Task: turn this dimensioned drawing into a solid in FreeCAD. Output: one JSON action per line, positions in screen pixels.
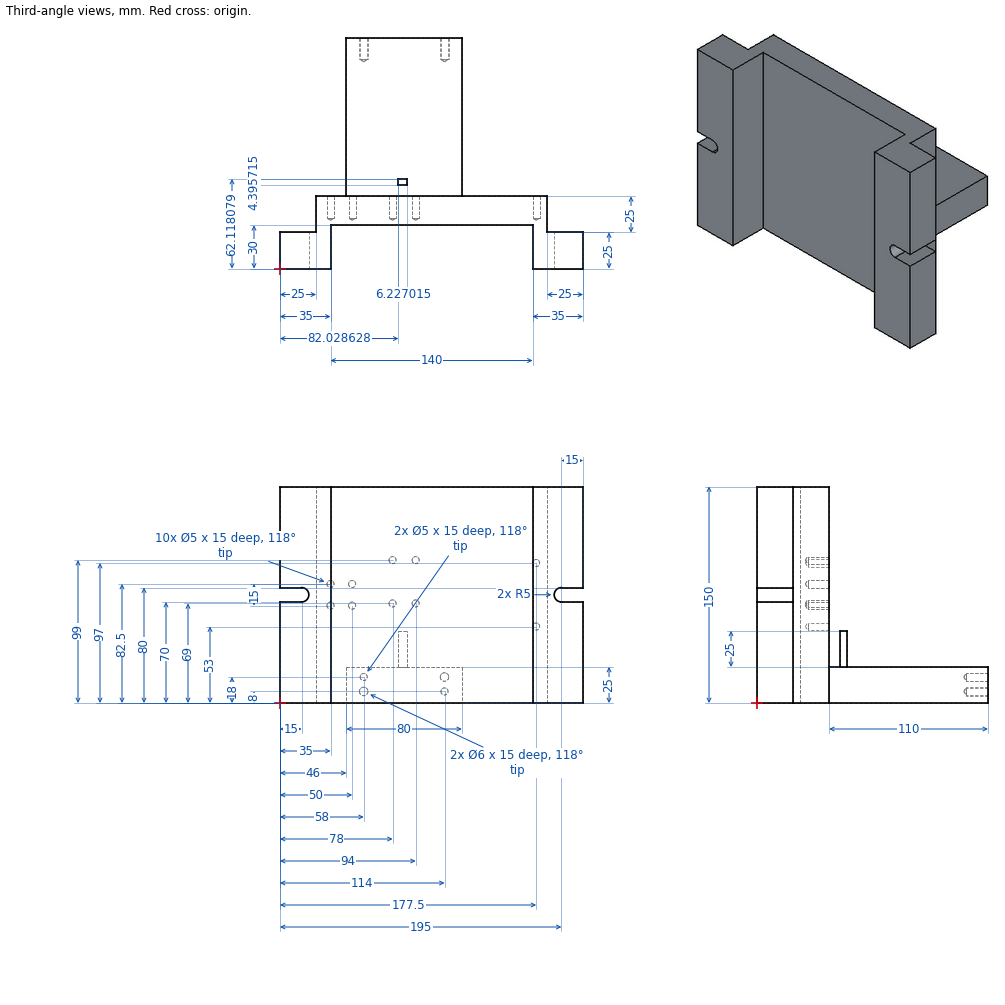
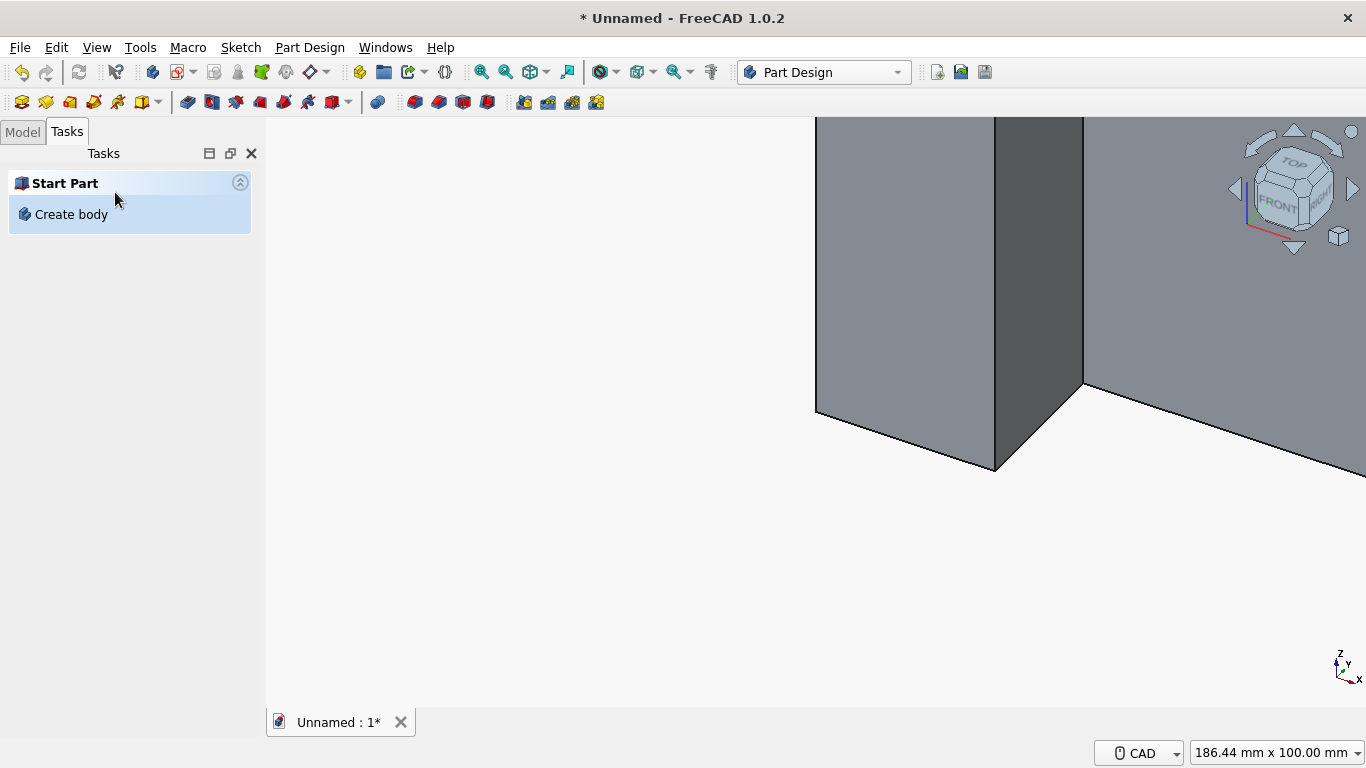
{"action": "left_click", "coordinate": [482, 72]}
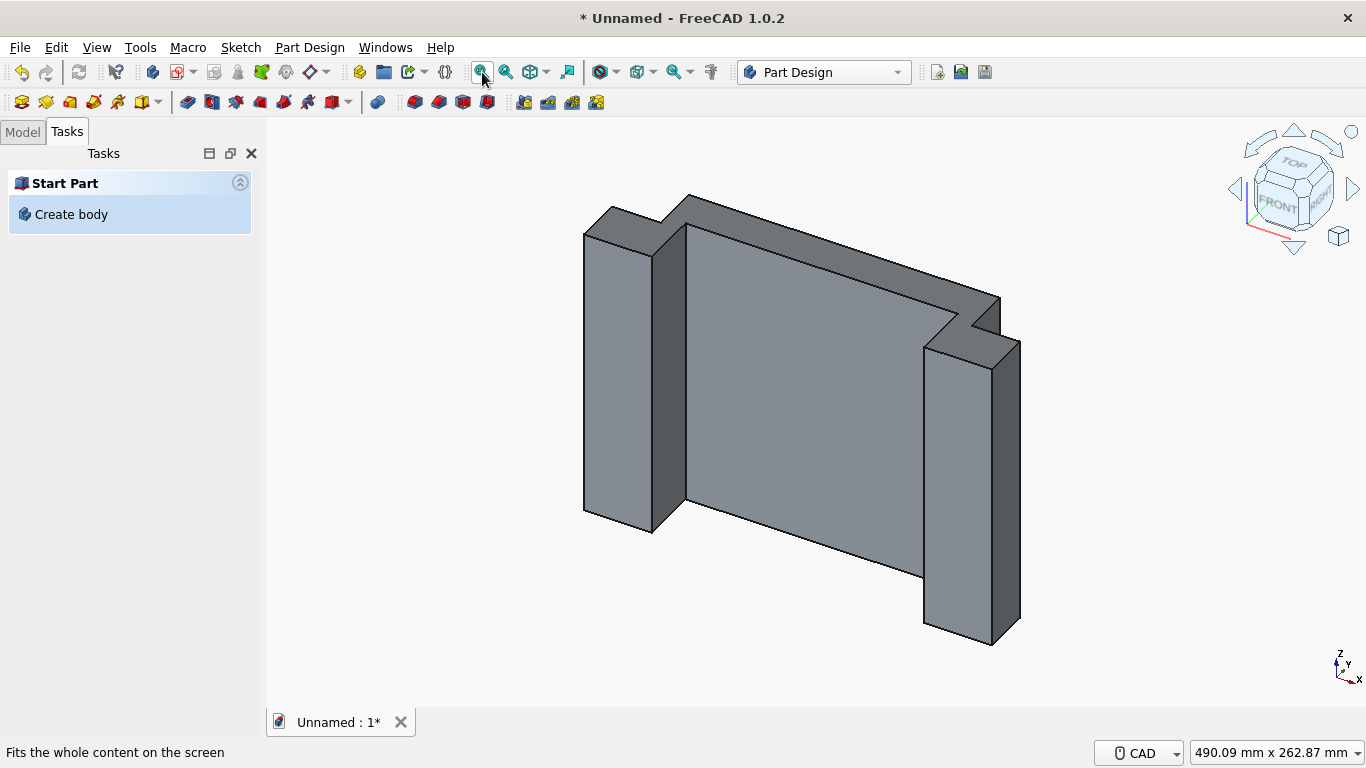
{"action": "key", "text": "4"}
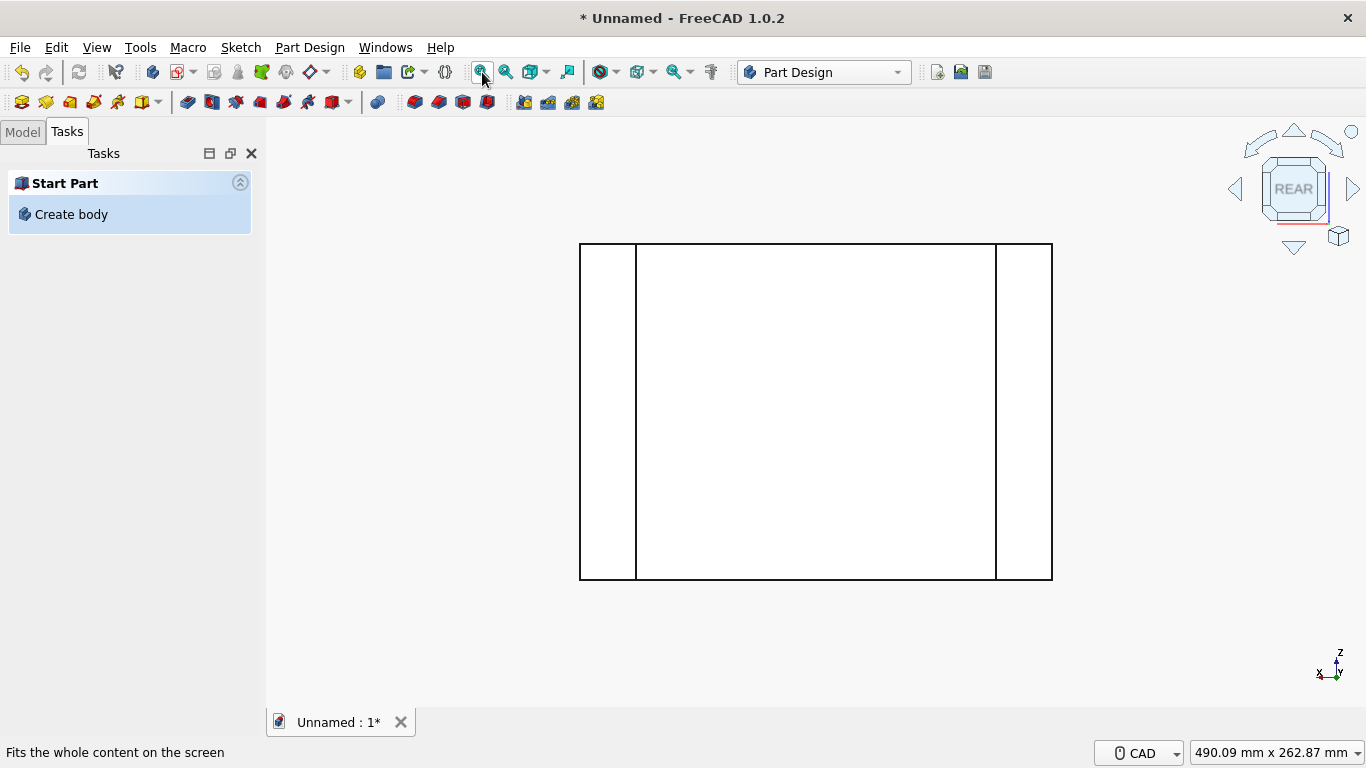
{"action": "left_click", "coordinate": [608, 315]}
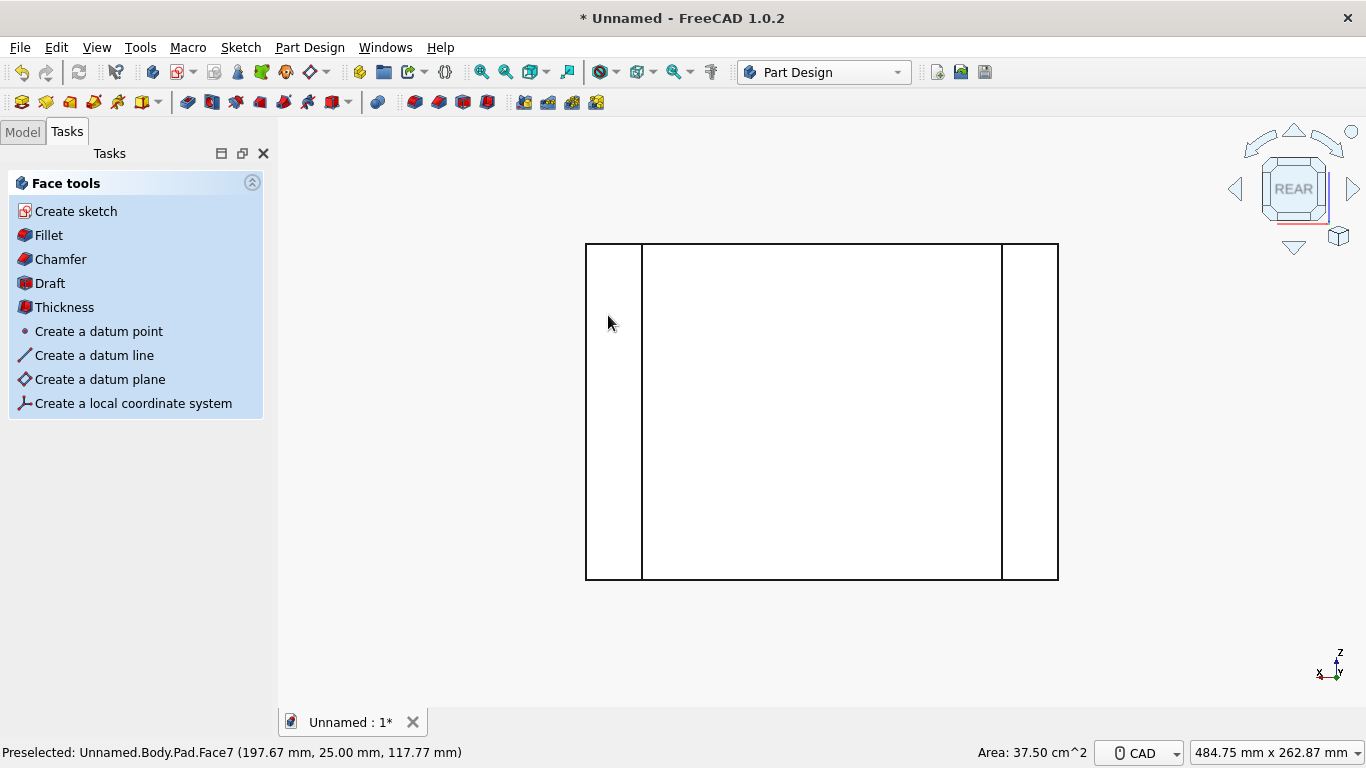
{"action": "left_click", "coordinate": [178, 72]}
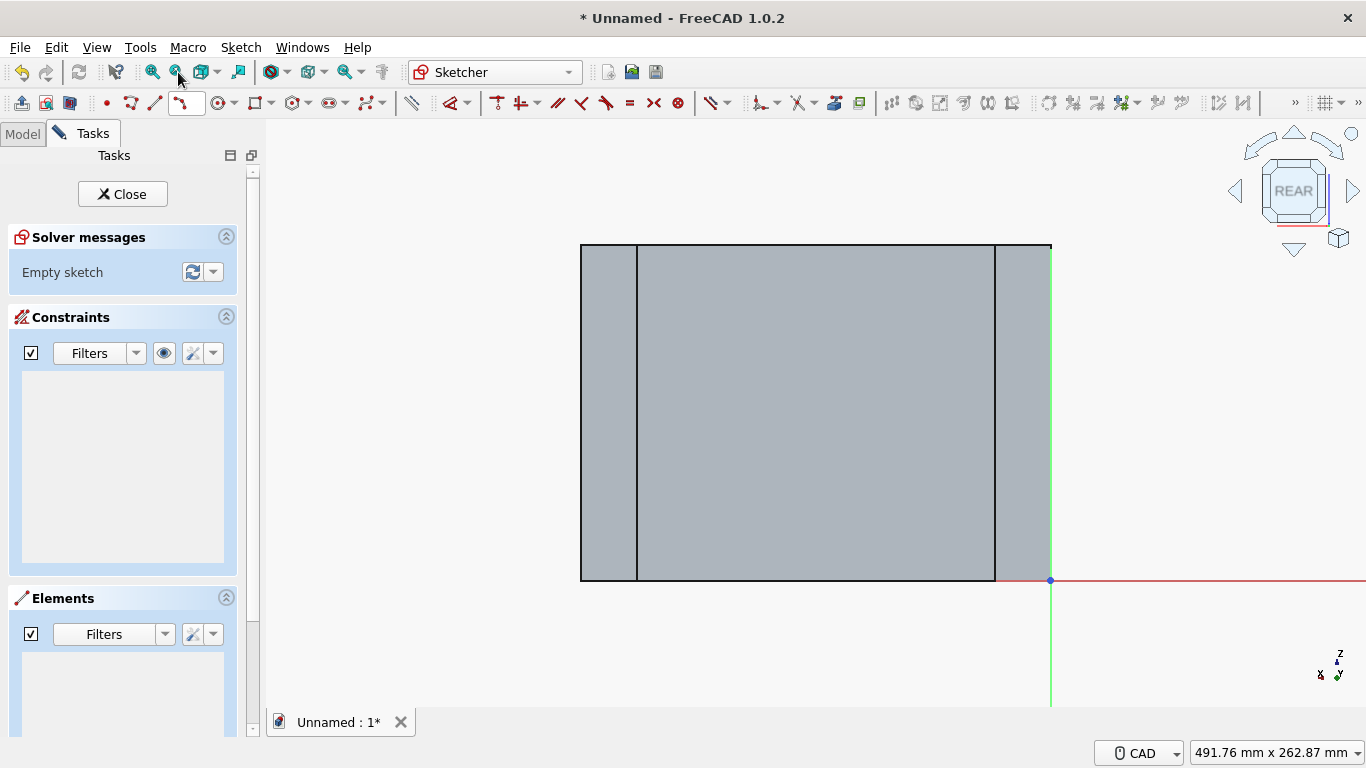
{"action": "scroll", "coordinate": [955, 650], "scroll_direction": "up", "scroll_amount": 2}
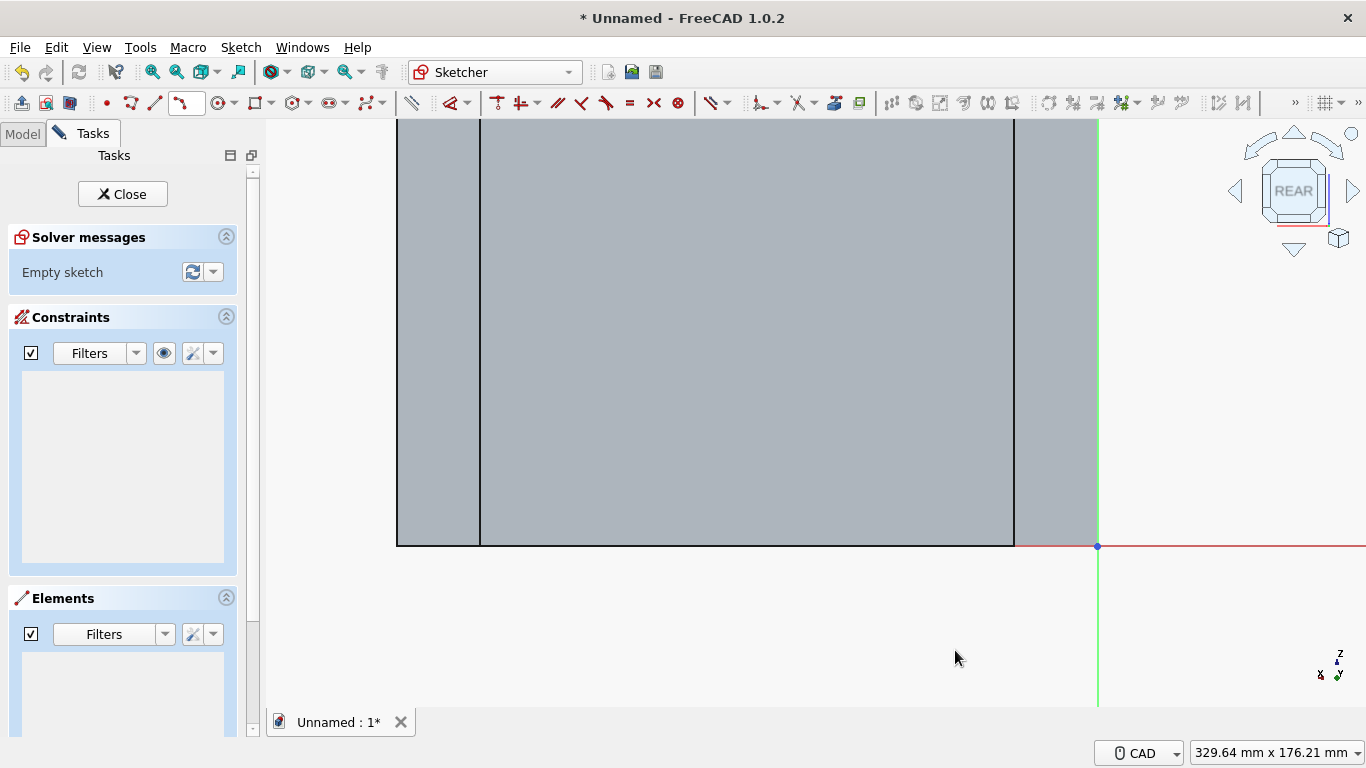
{"action": "left_click", "coordinate": [132, 104]}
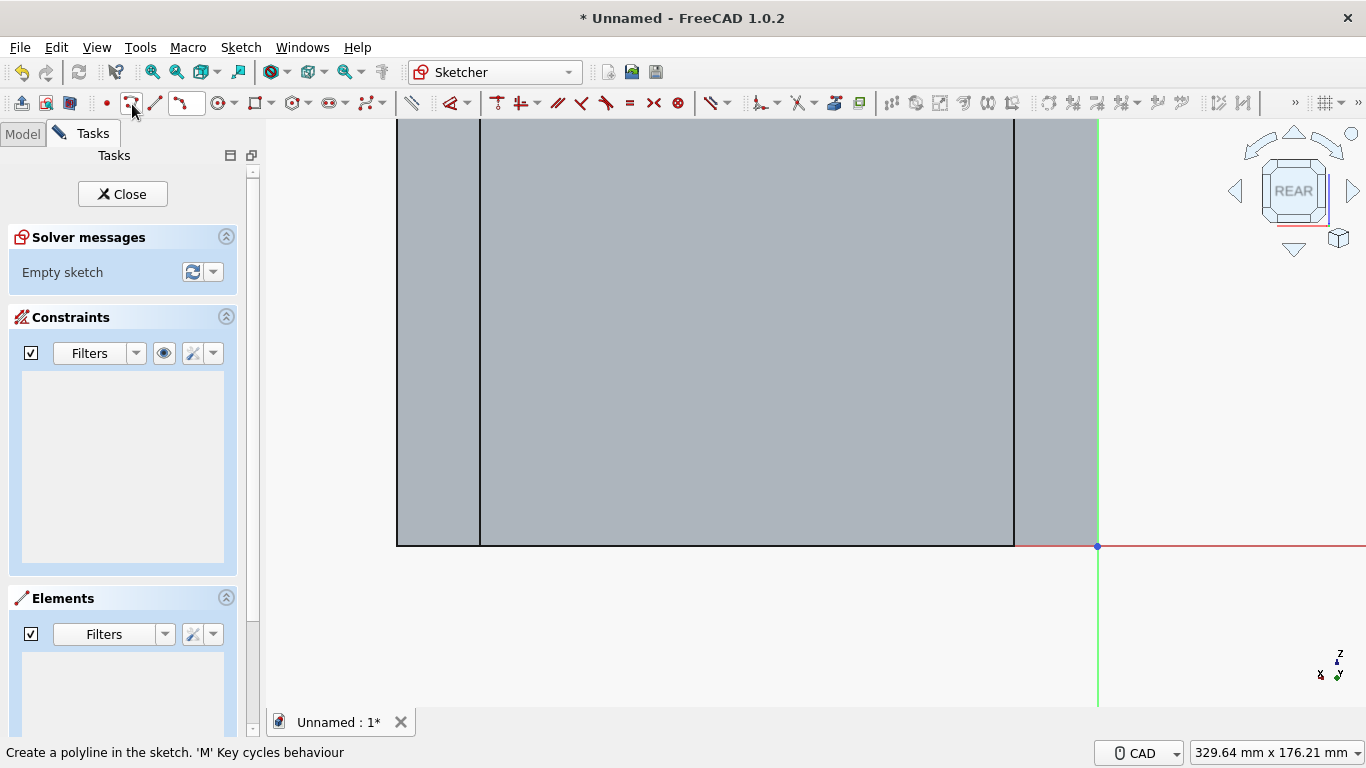
{"action": "left_click", "coordinate": [447, 279]}
{"action": "left_click", "coordinate": [397, 279]}
{"action": "left_click", "coordinate": [397, 313]}
{"action": "left_click", "coordinate": [447, 313]}
{"action": "right_click", "coordinate": [447, 313]}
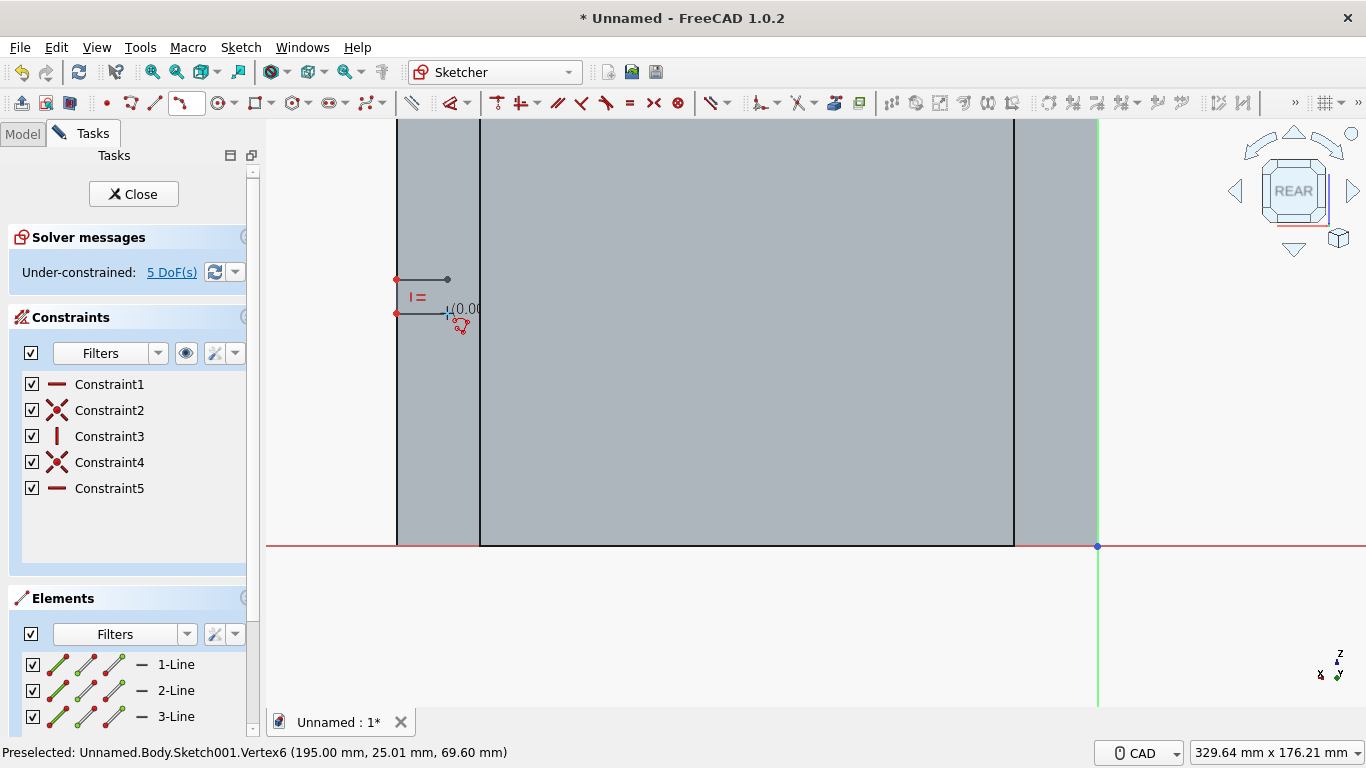
{"action": "left_click", "coordinate": [180, 104]}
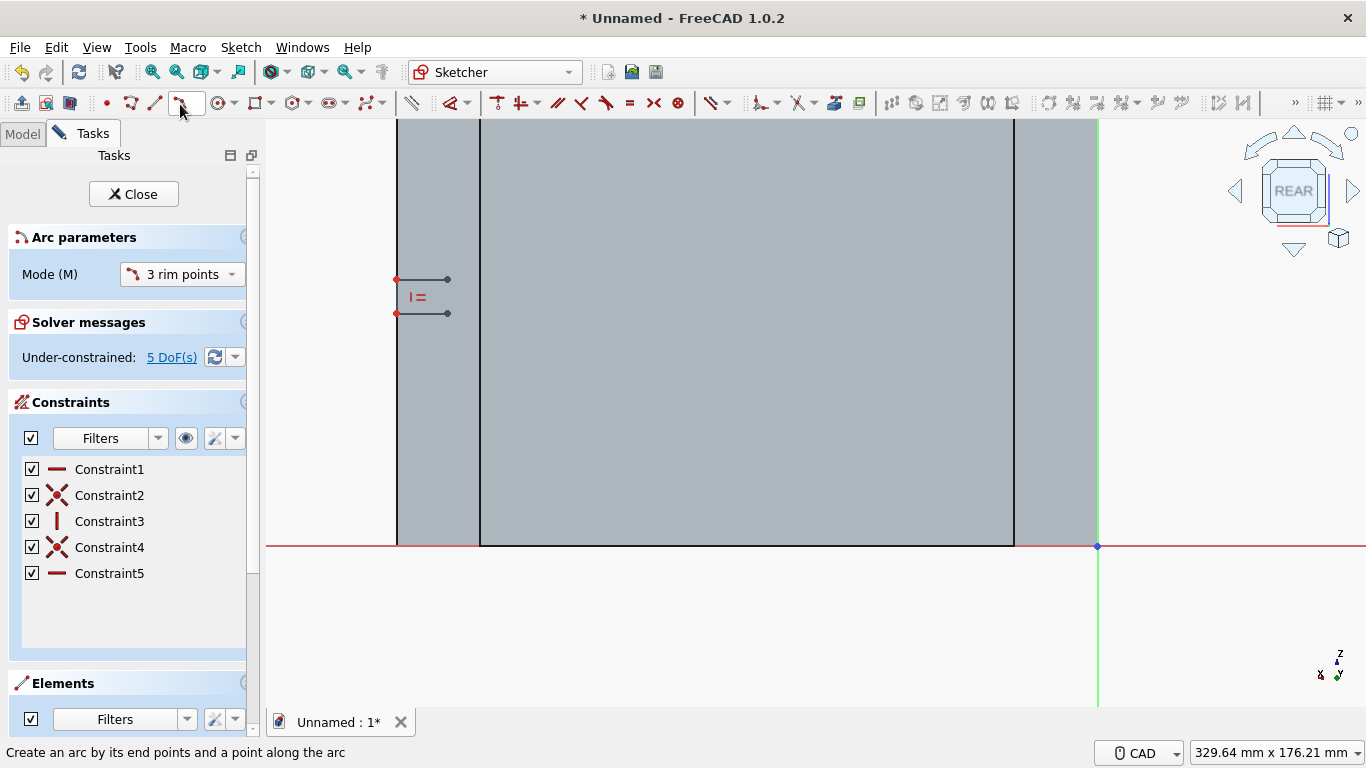
{"action": "left_click", "coordinate": [447, 314]}
{"action": "left_click", "coordinate": [447, 280]}
{"action": "left_click", "coordinate": [464, 296]}